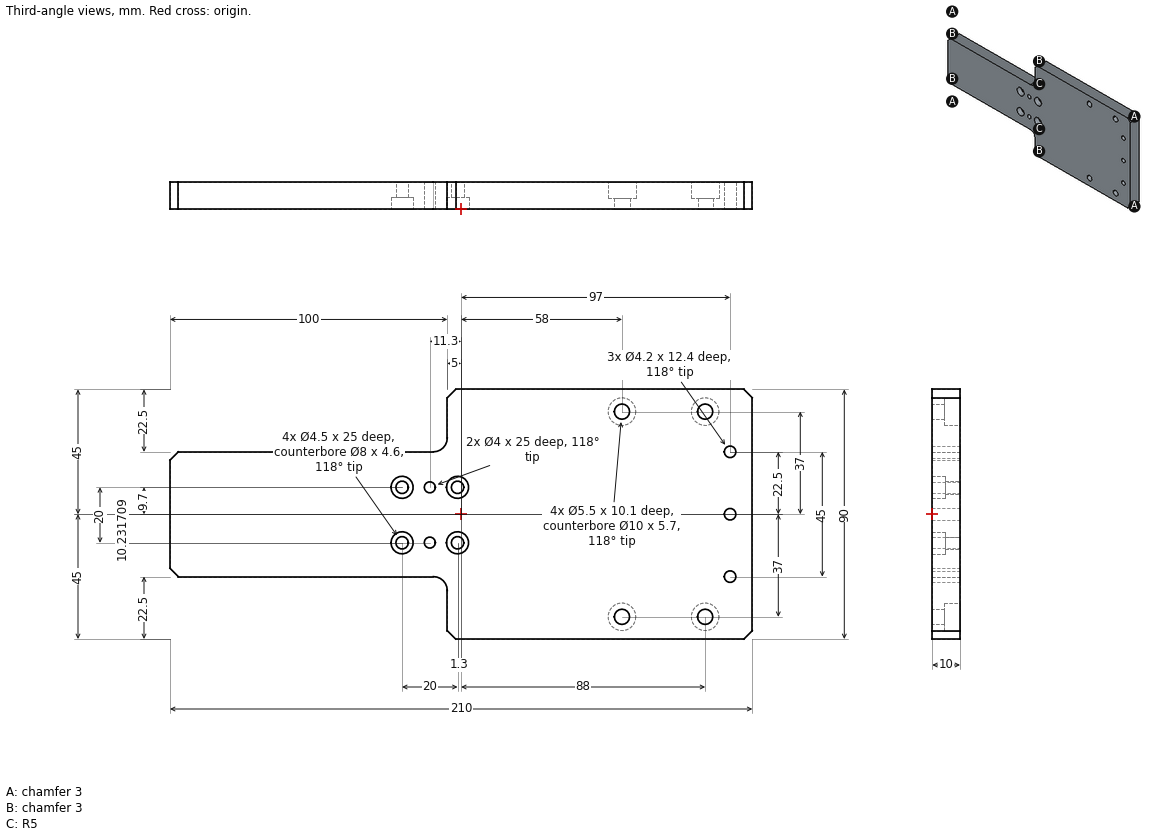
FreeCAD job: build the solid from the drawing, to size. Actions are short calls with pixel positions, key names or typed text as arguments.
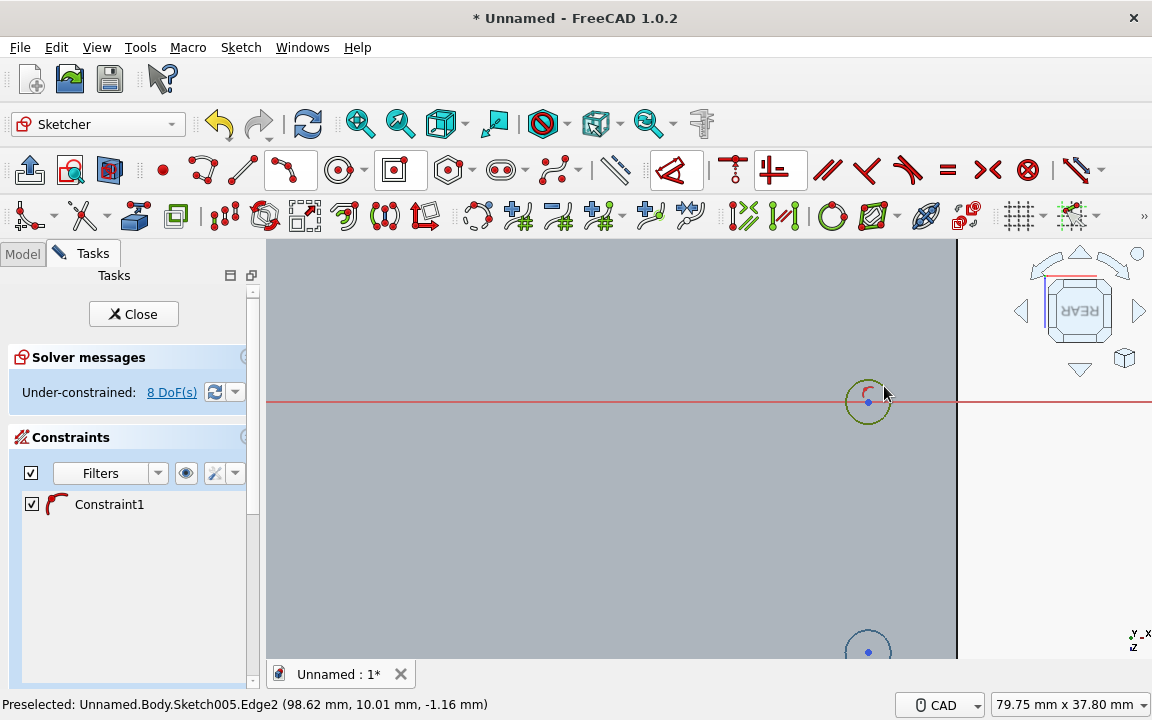
scroll(885, 487, down, 4)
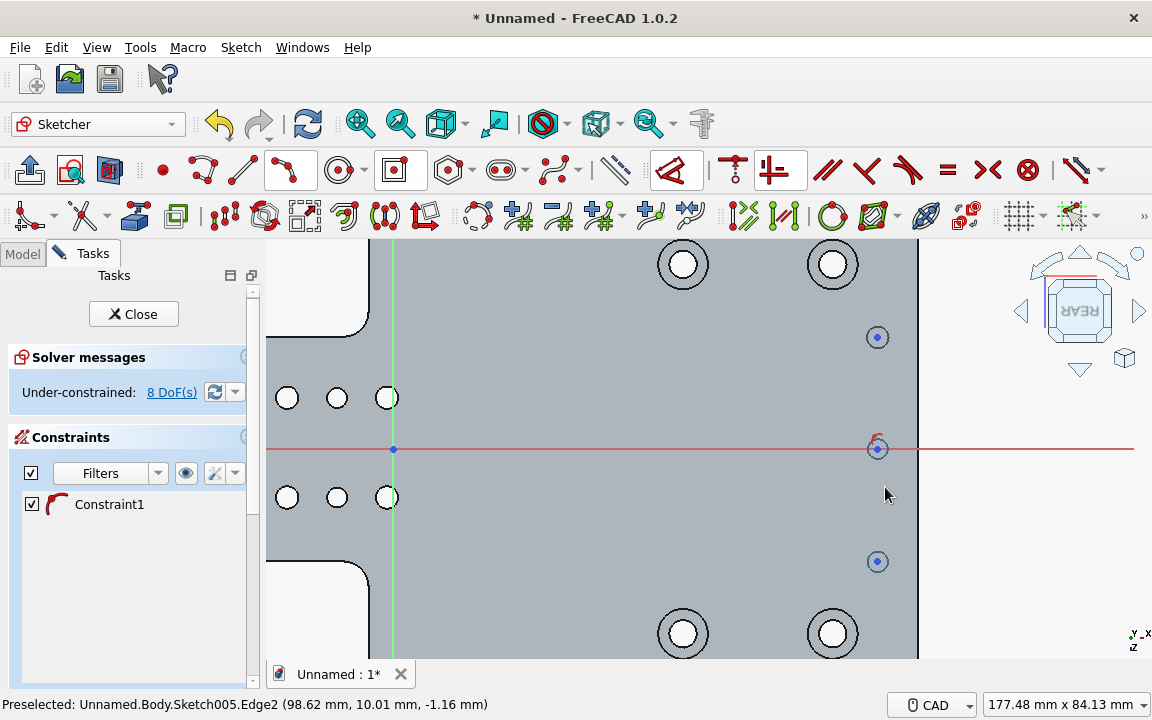
scroll(885, 330, up, 2)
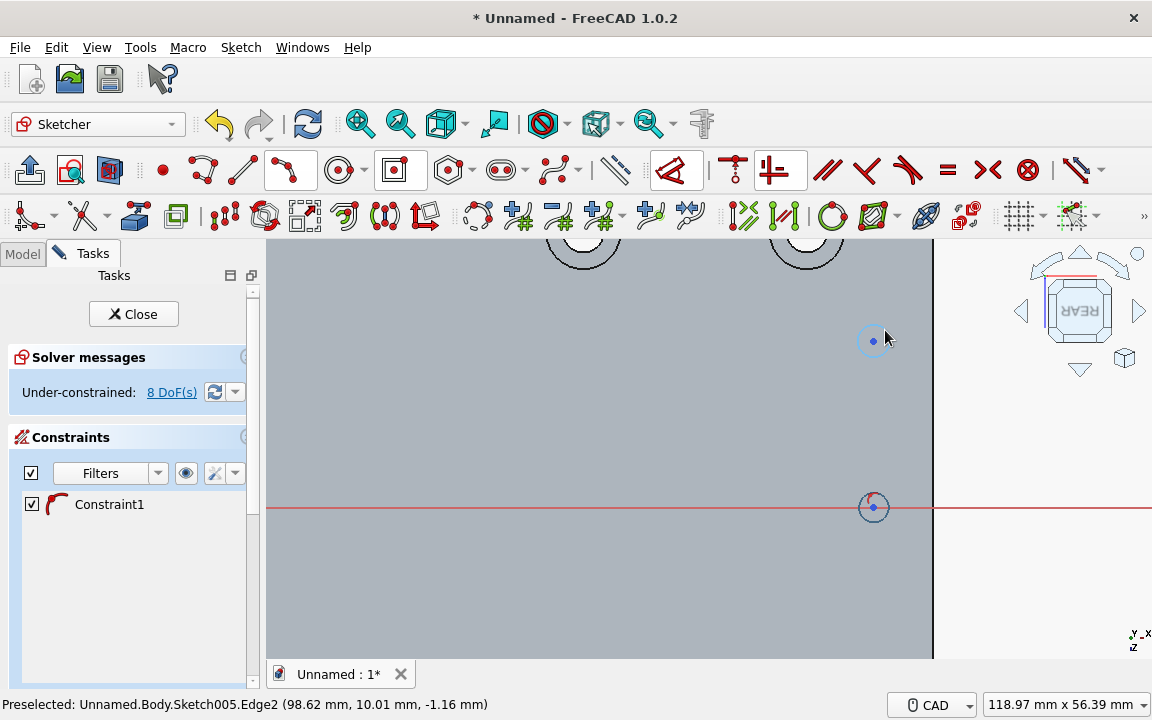
click(885, 330)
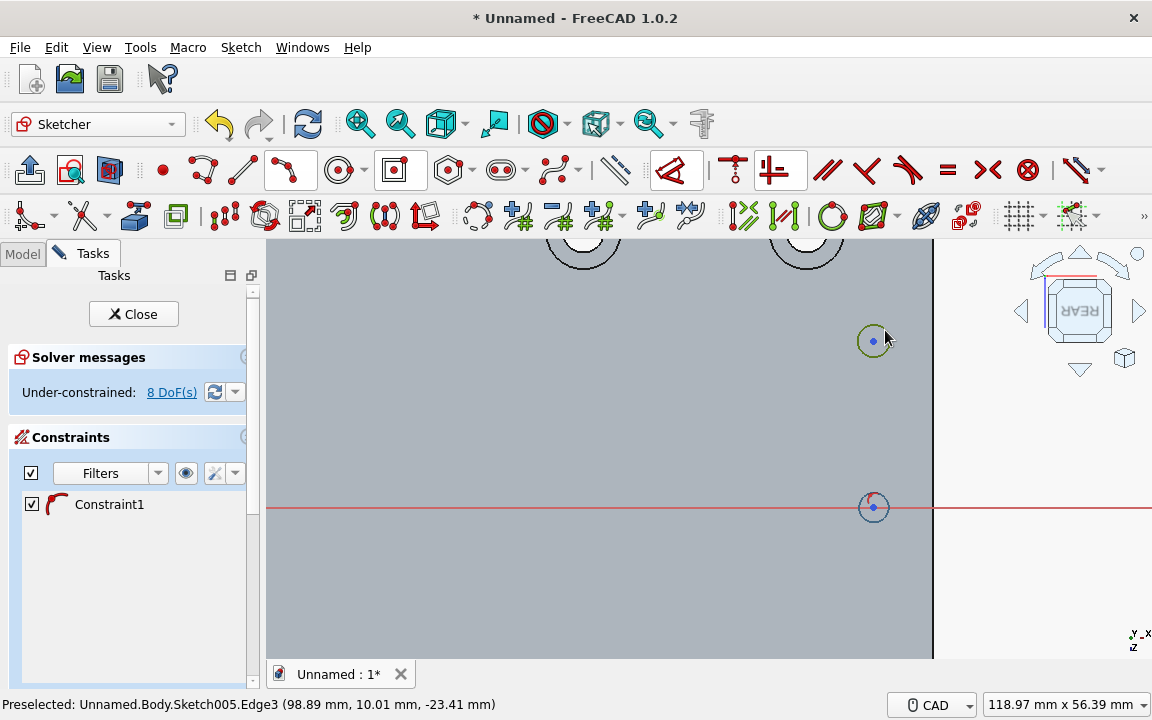
click(948, 170)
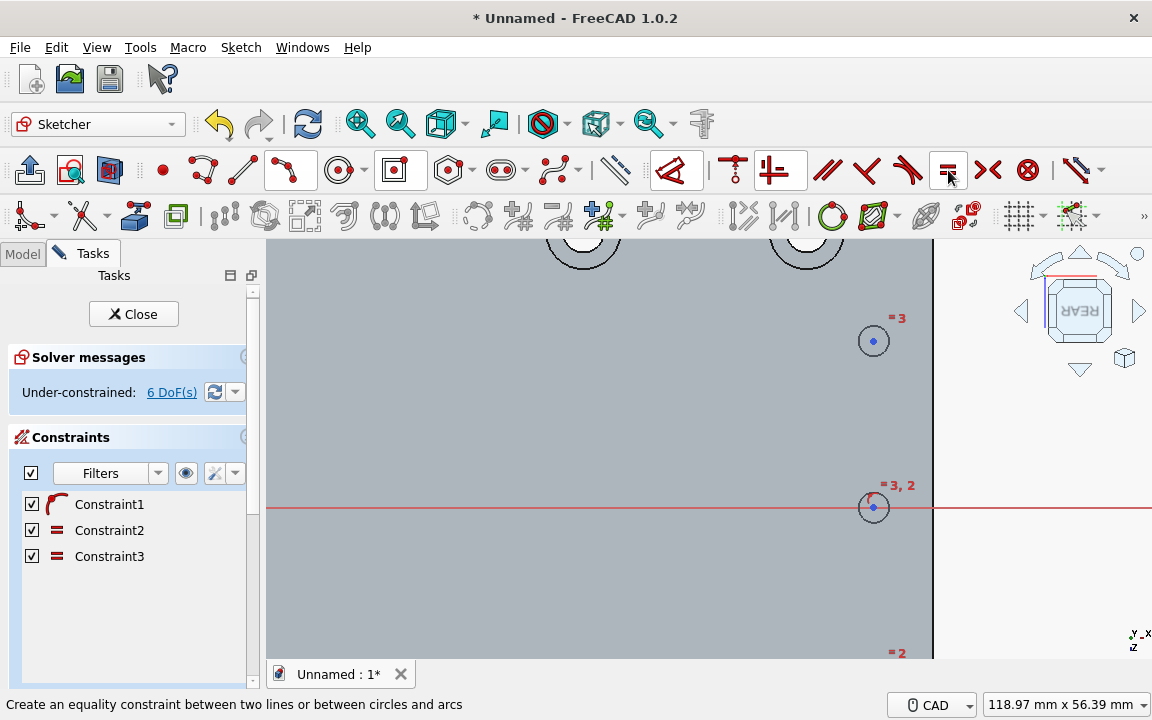
scroll(885, 330, down, 2)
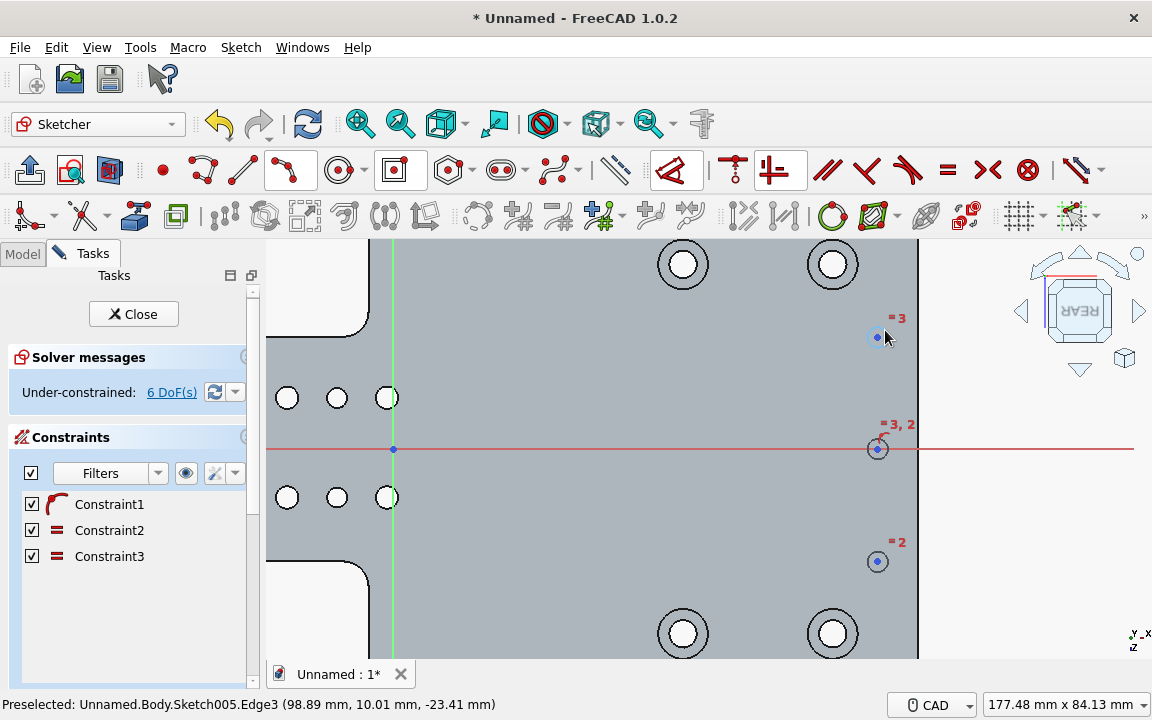
click(878, 562)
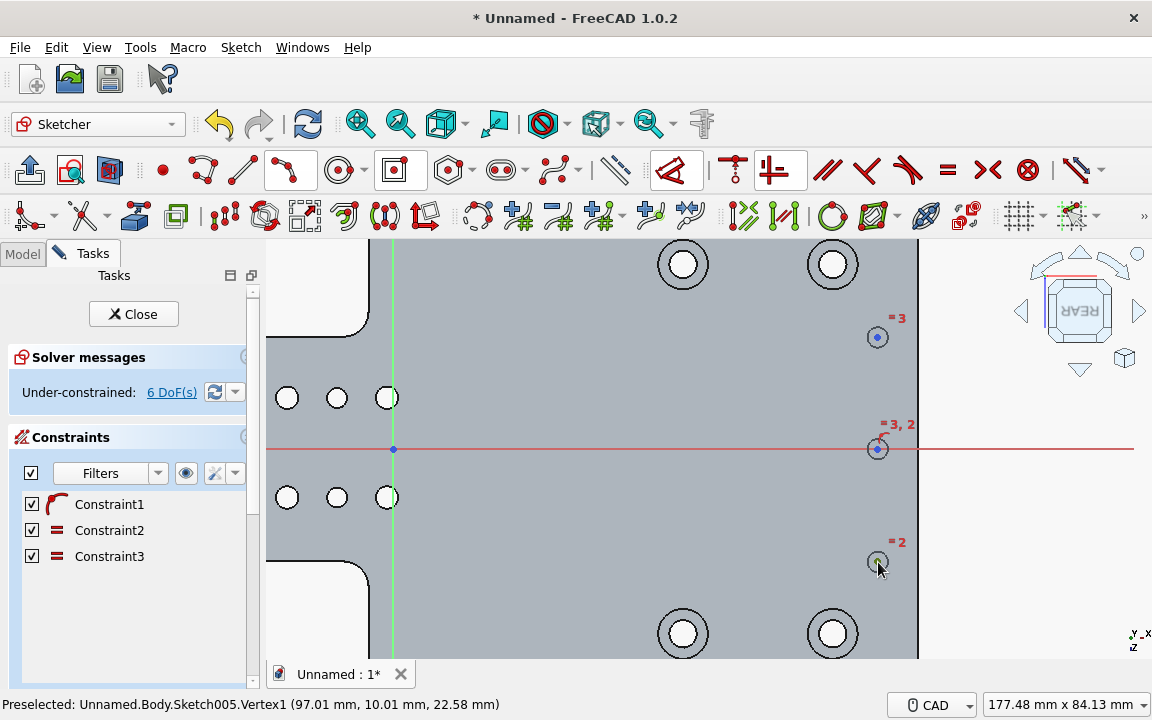
click(878, 449)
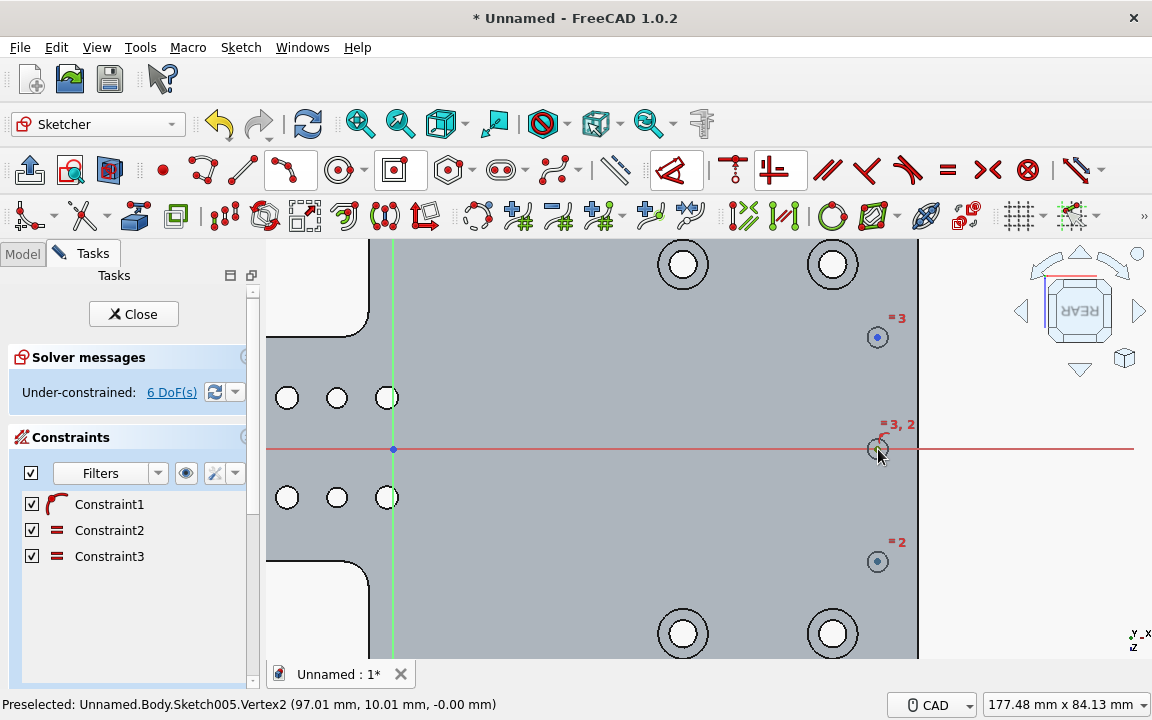
click(802, 170)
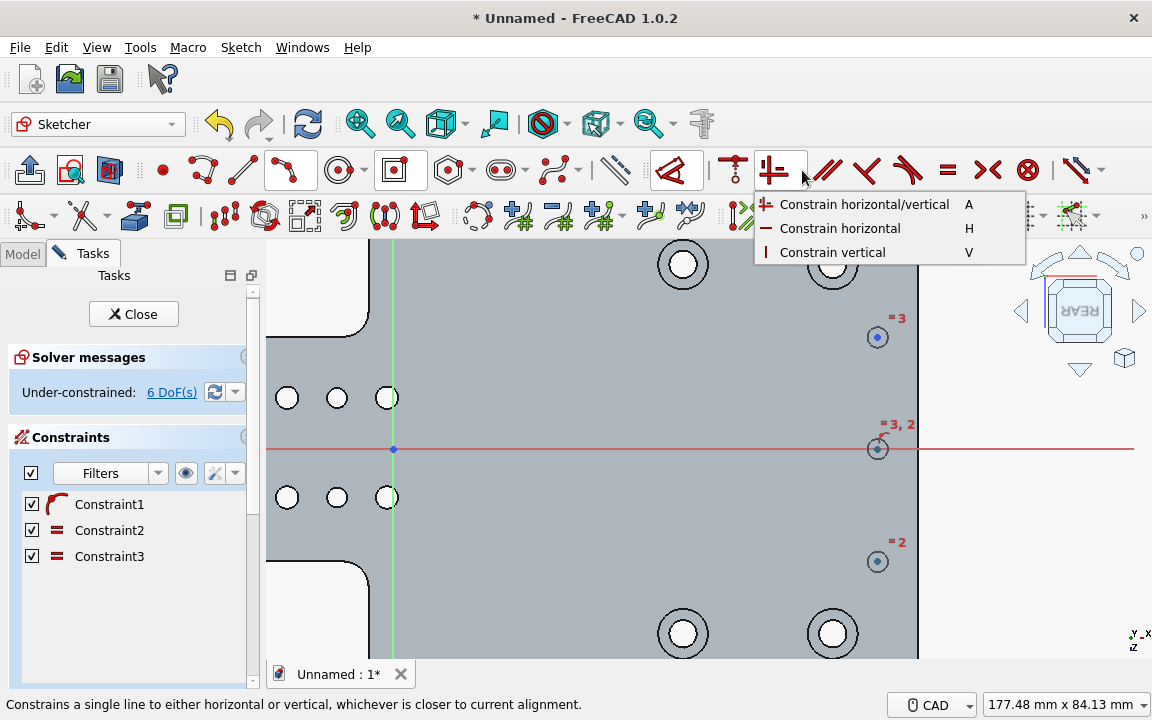
click(890, 252)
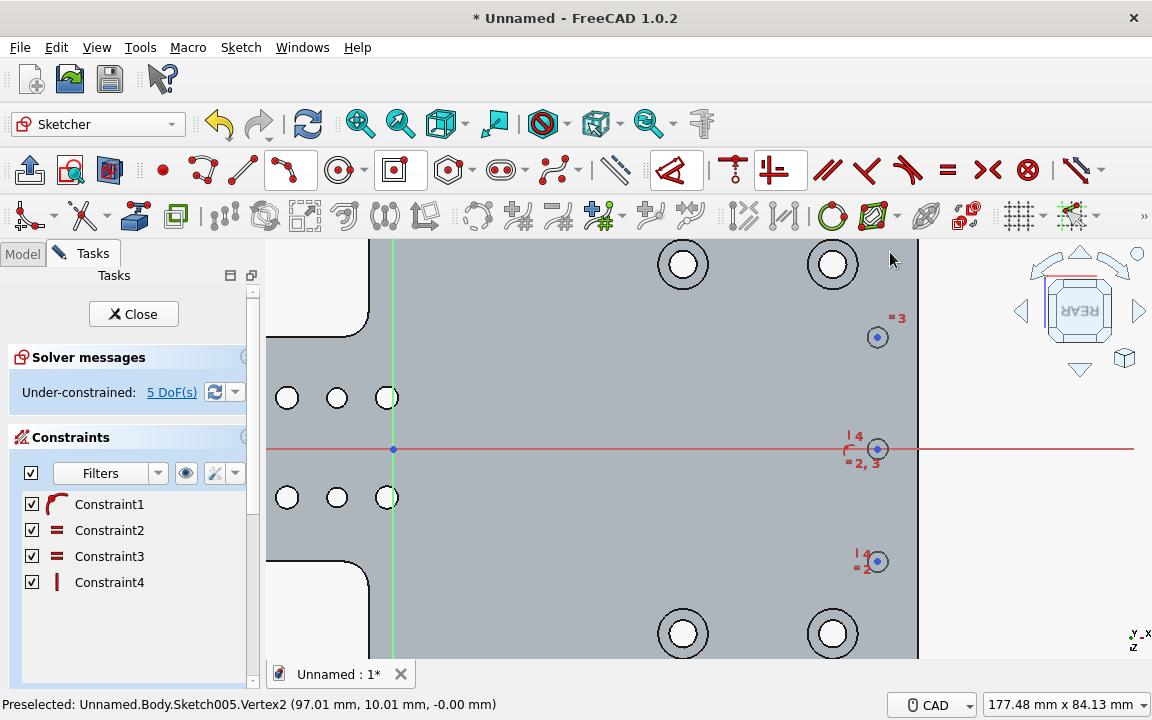
click(880, 451)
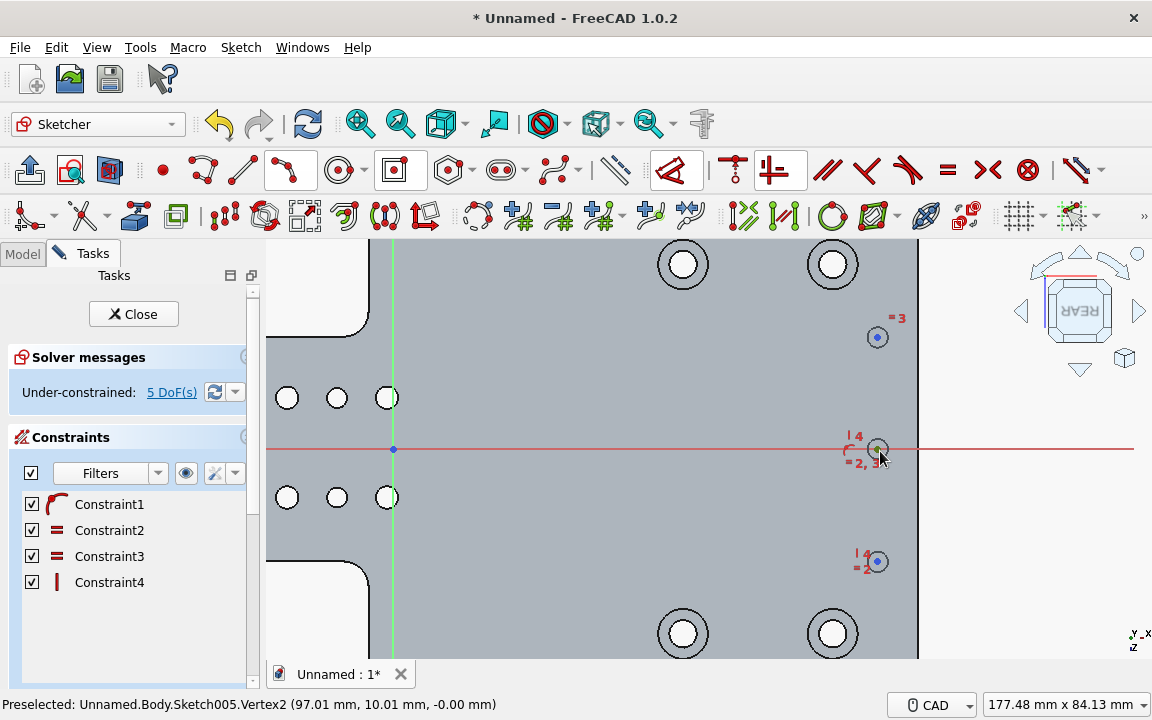
click(878, 337)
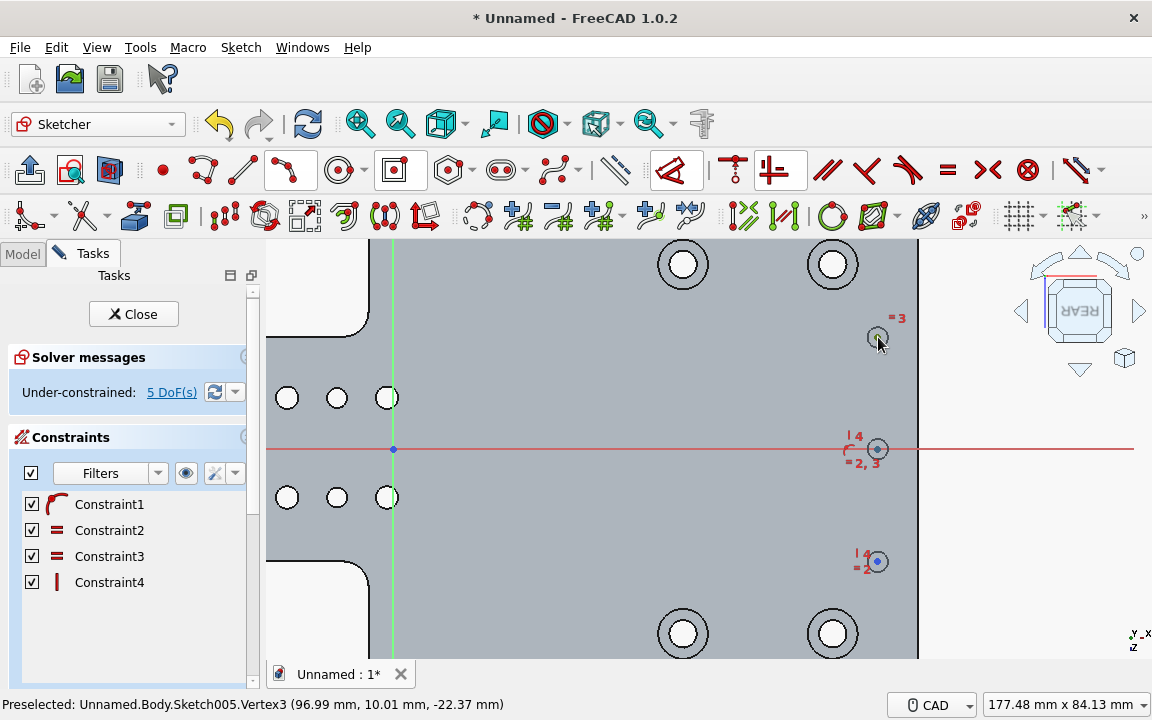
key(v)